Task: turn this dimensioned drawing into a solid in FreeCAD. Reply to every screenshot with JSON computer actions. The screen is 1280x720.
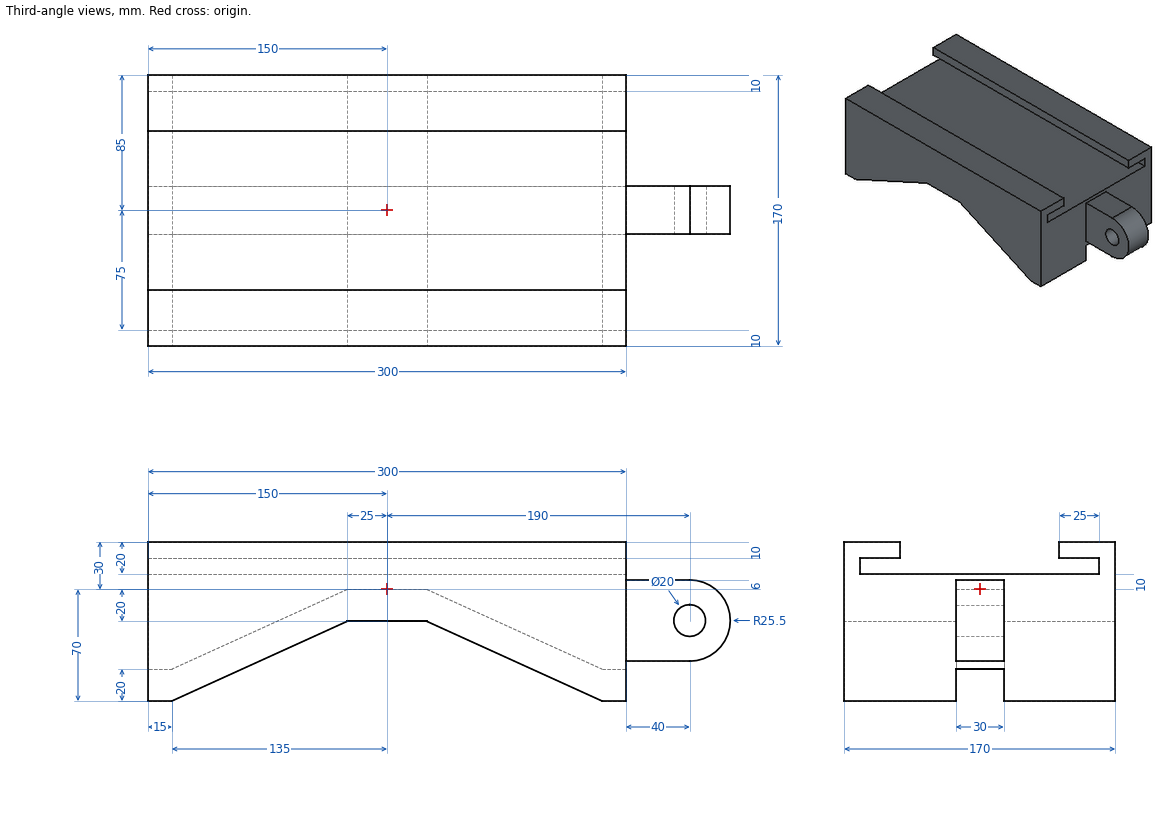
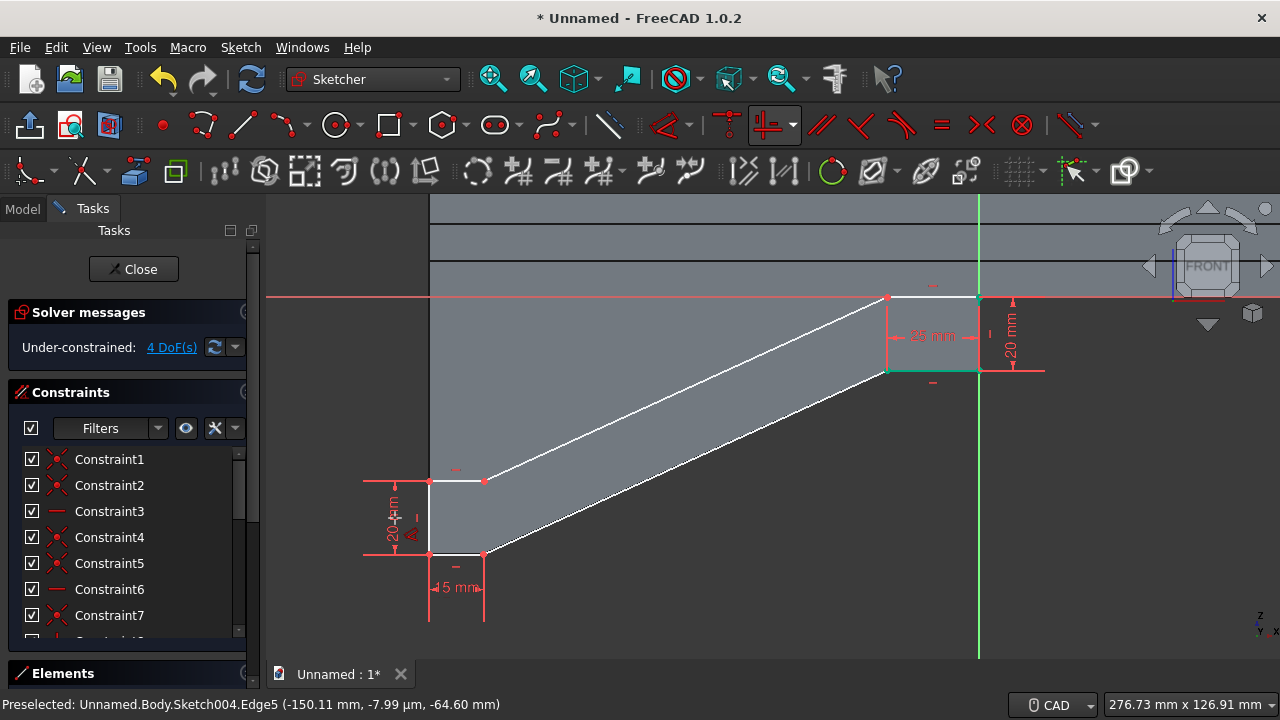
{"action": "left_click", "coordinate": [445, 481]}
{"action": "left_click", "coordinate": [469, 515]}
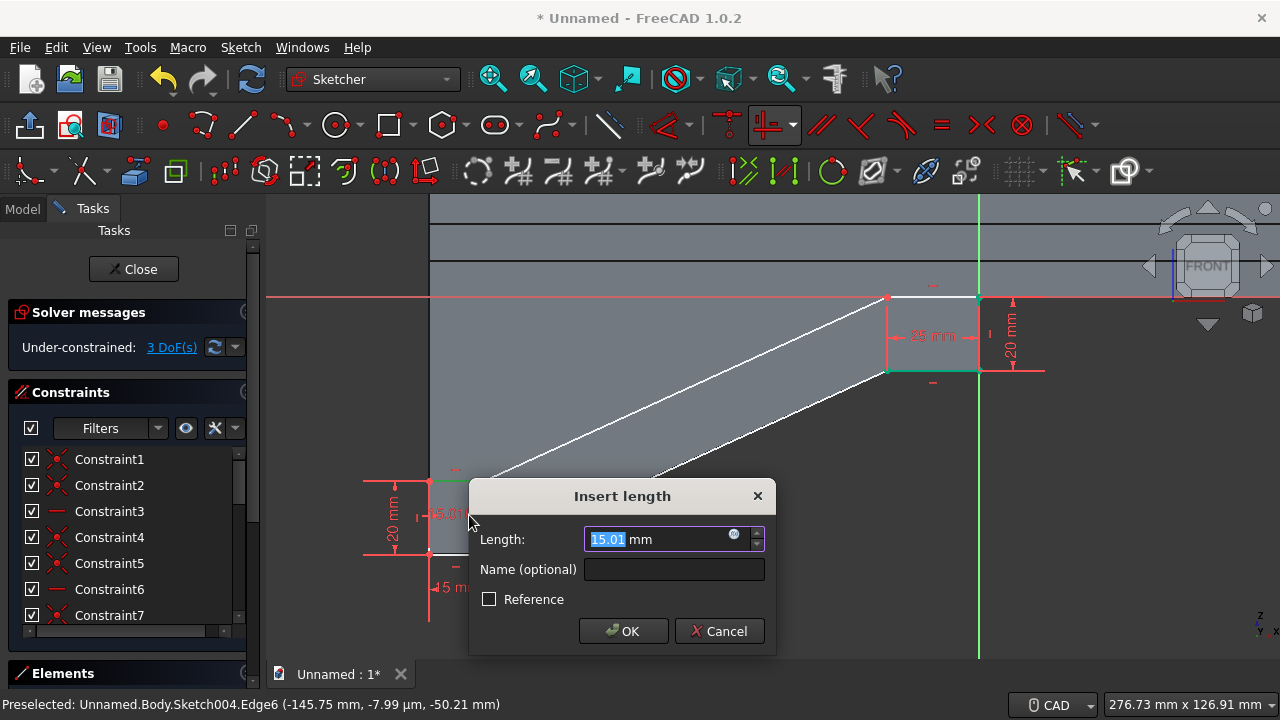
{"action": "type", "text": "15"}
{"action": "key", "text": "Return"}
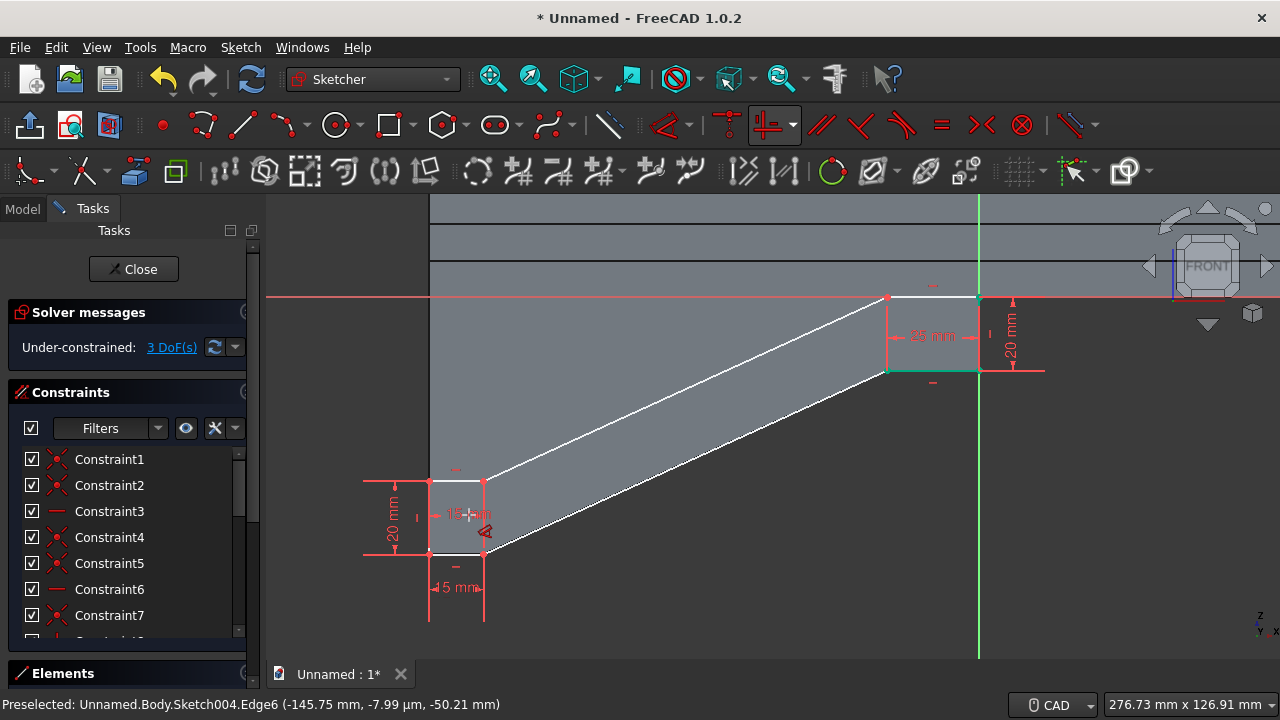
{"action": "left_click", "coordinate": [915, 297]}
{"action": "left_click", "coordinate": [933, 263]}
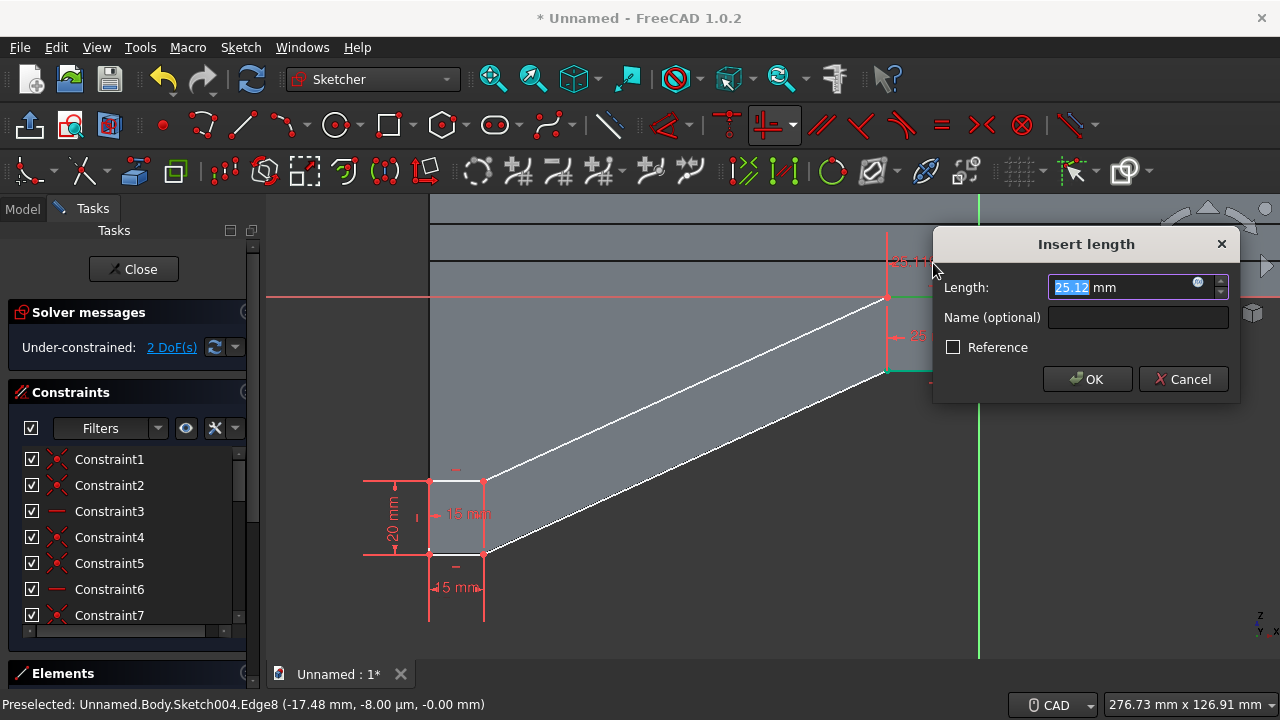
{"action": "type", "text": "25"}
{"action": "key", "text": "Return"}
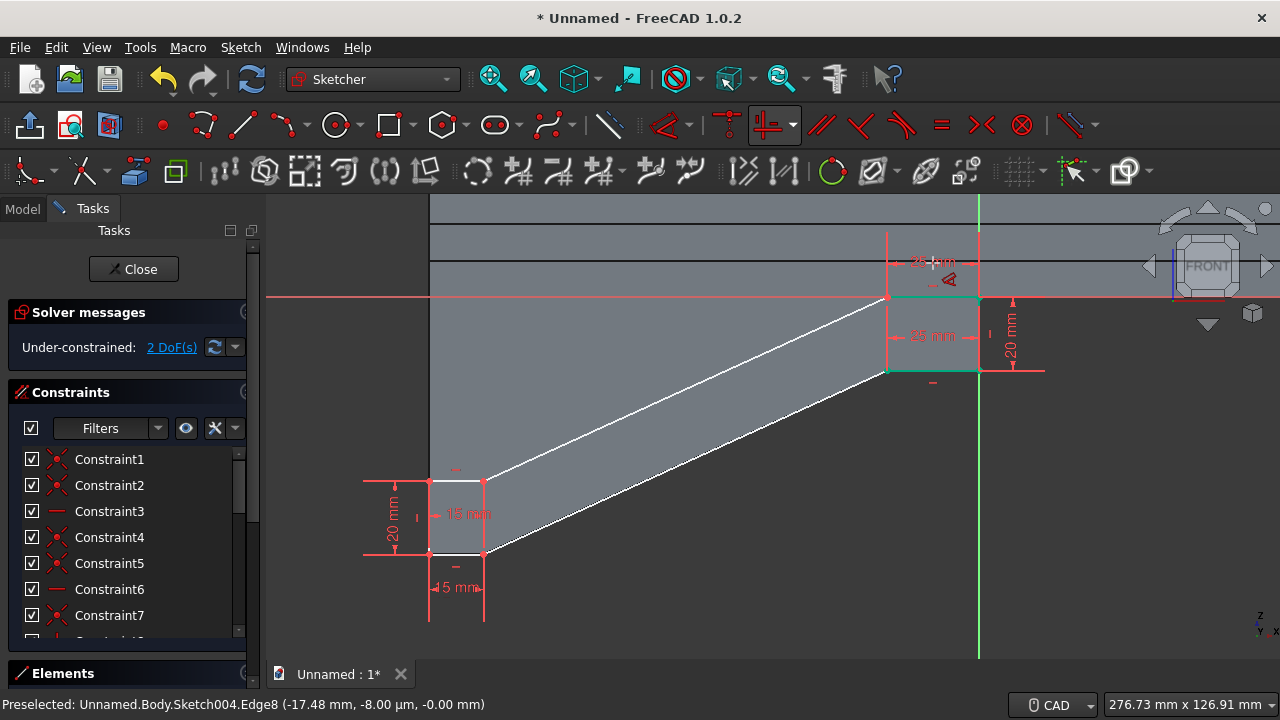
{"action": "left_click", "coordinate": [484, 555]}
{"action": "left_click", "coordinate": [1013, 426]}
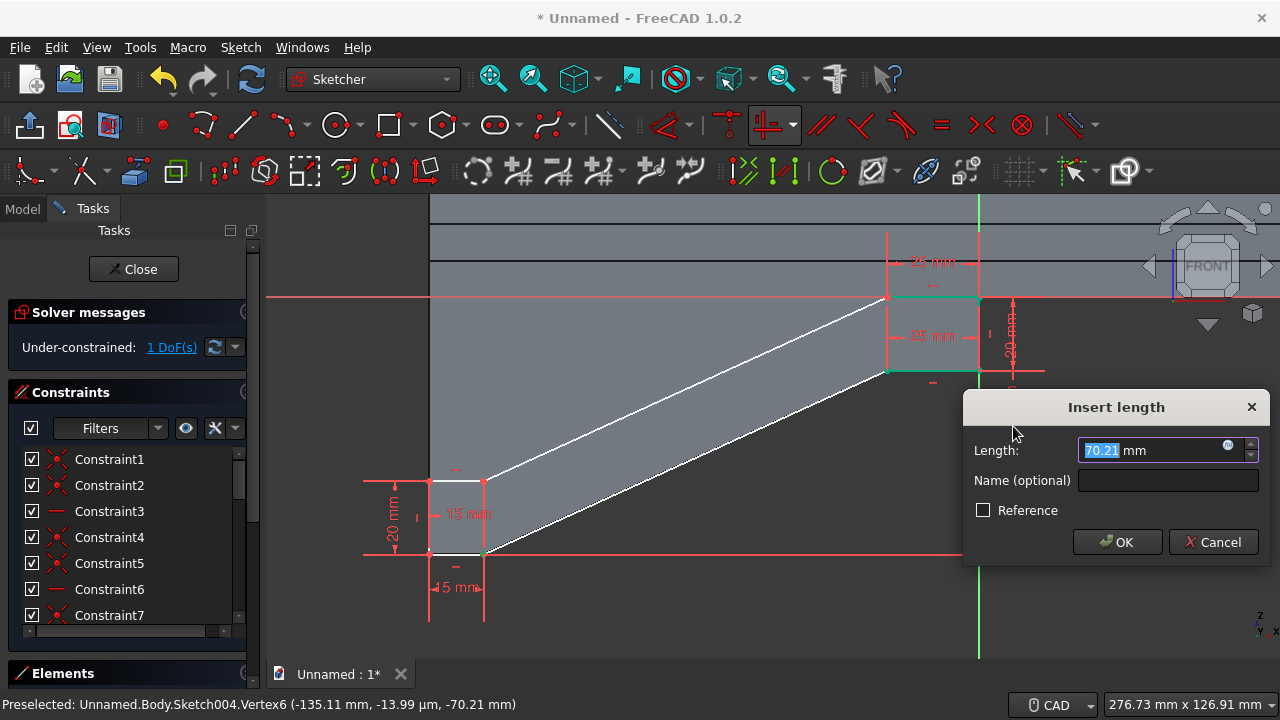
{"action": "type", "text": "70"}
{"action": "key", "text": "Return"}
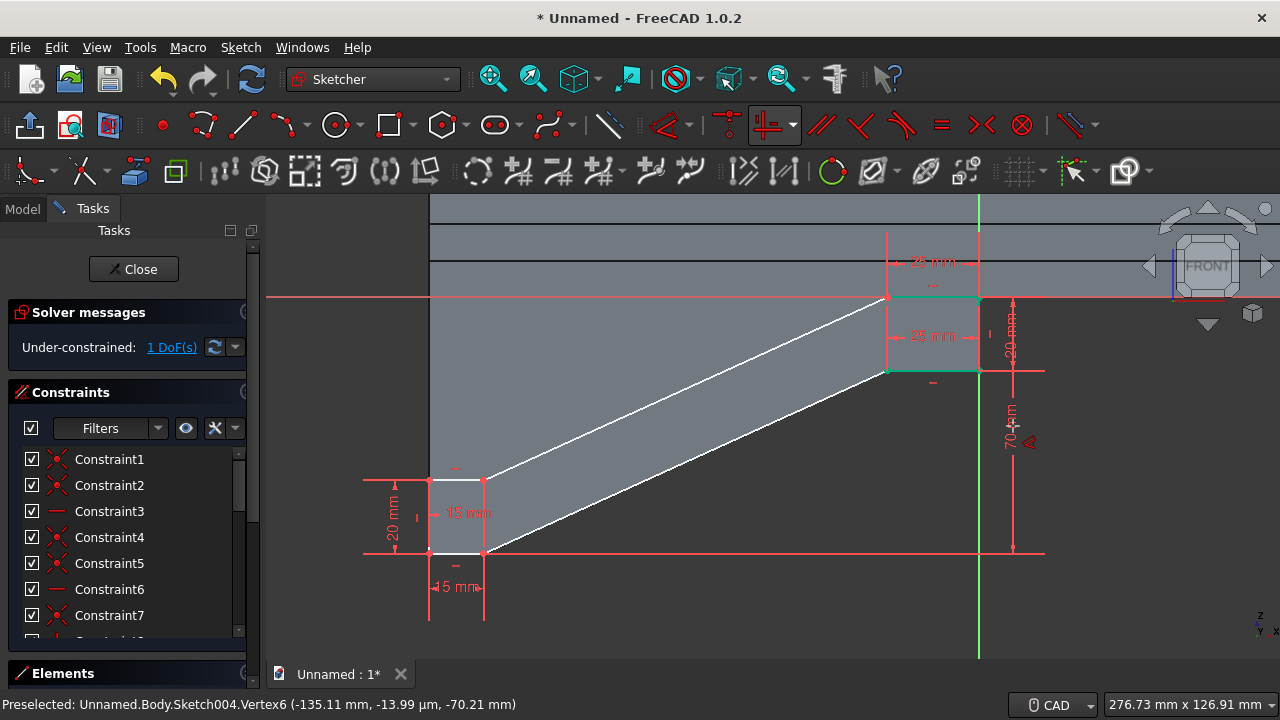
{"action": "left_click", "coordinate": [484, 554]}
{"action": "left_click", "coordinate": [732, 588]}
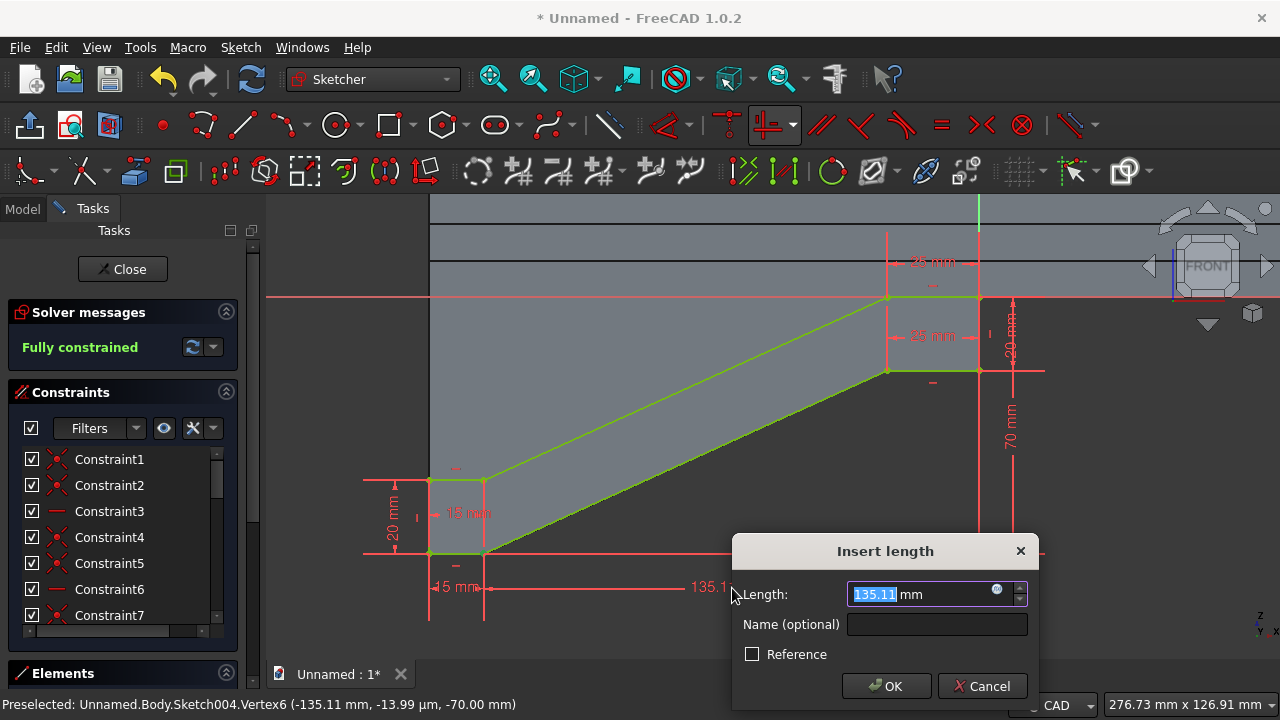
{"action": "type", "text": "135"}
{"action": "key", "text": "Return"}
{"action": "key", "text": "Escape"}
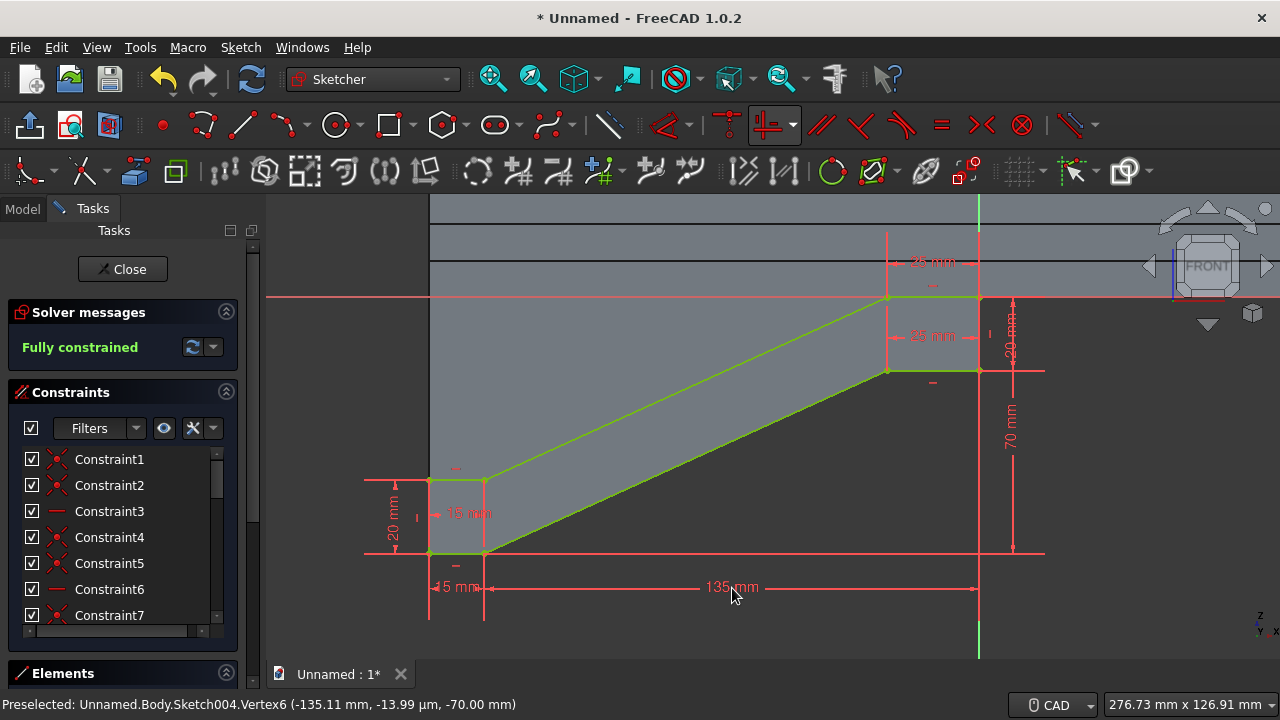
{"action": "left_click", "coordinate": [123, 269]}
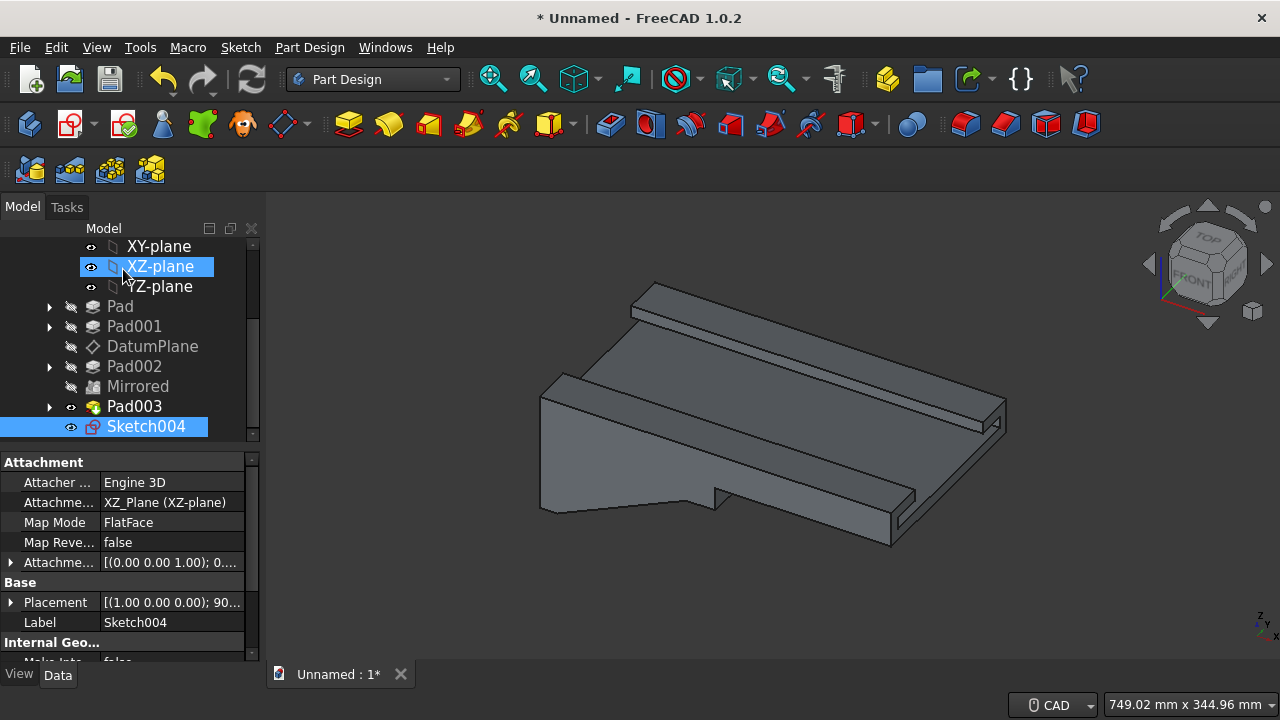
{"action": "left_click", "coordinate": [612, 124]}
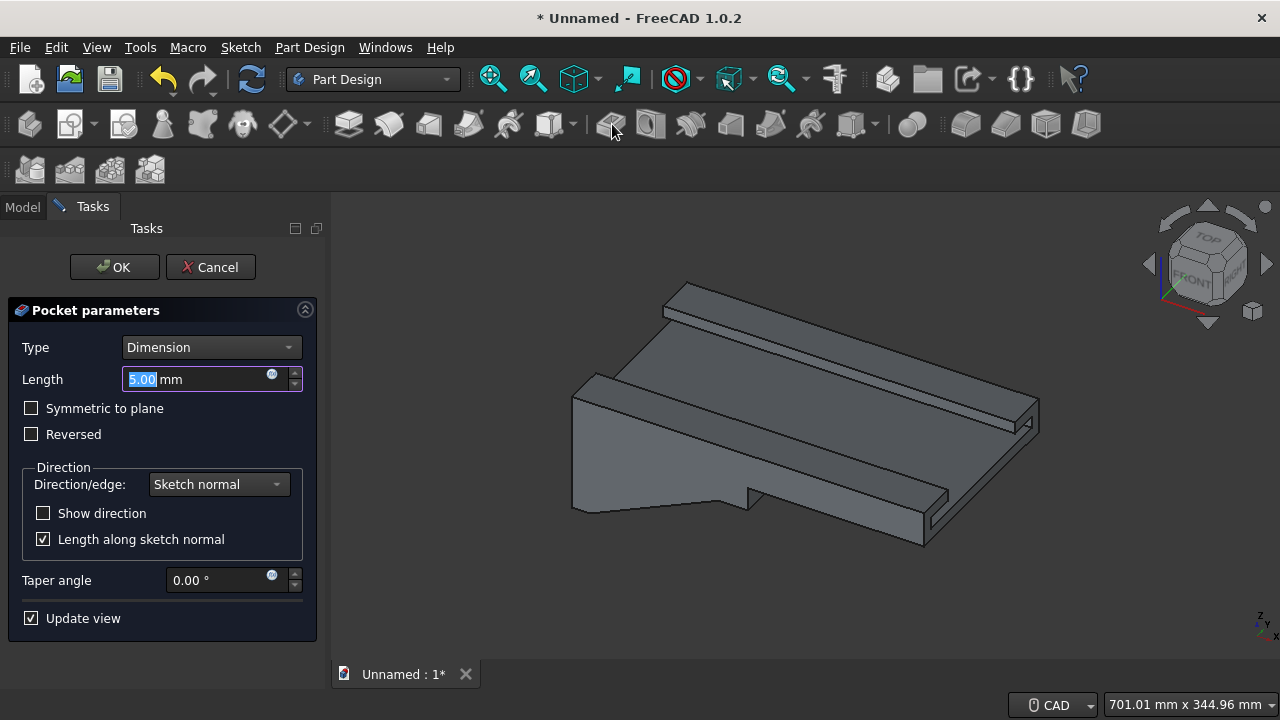
{"action": "type", "text": "30"}
{"action": "key", "text": "Tab"}